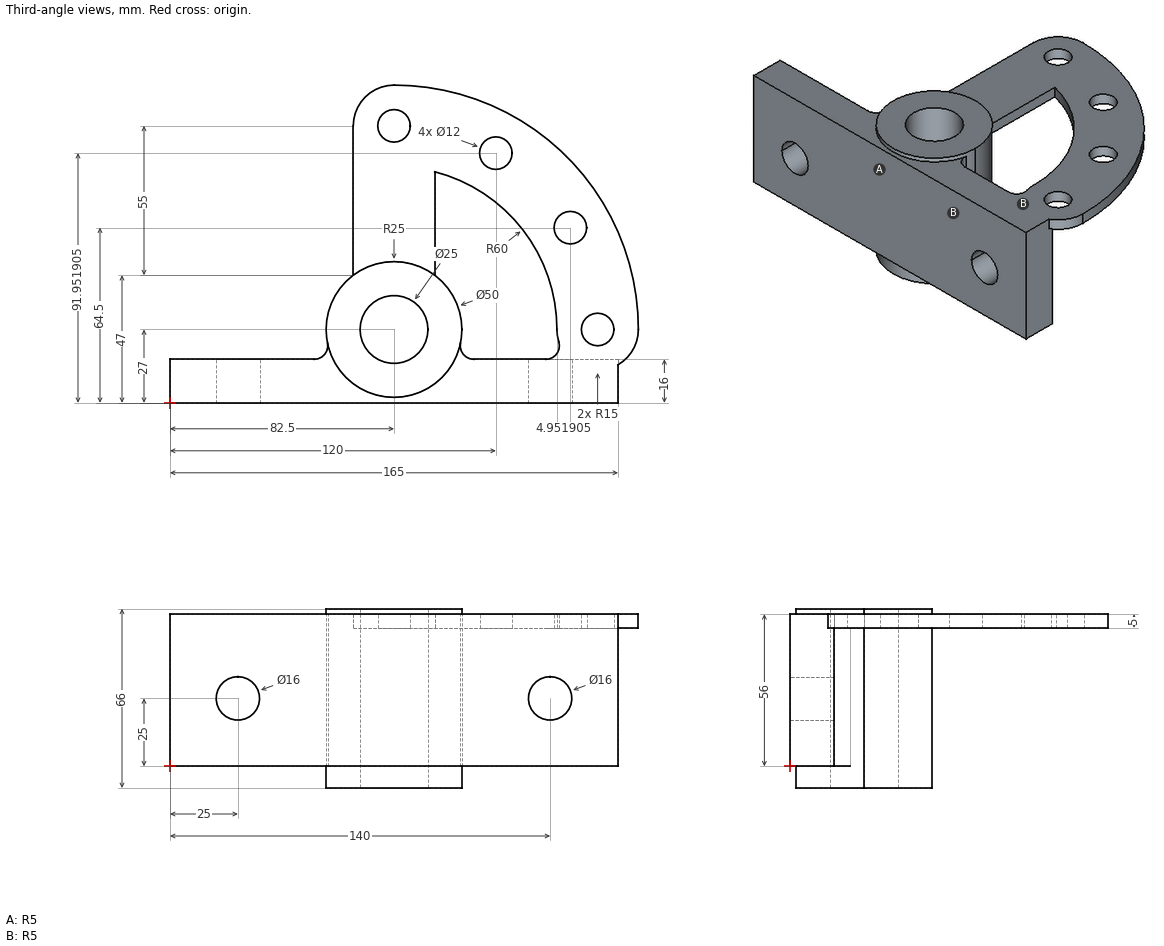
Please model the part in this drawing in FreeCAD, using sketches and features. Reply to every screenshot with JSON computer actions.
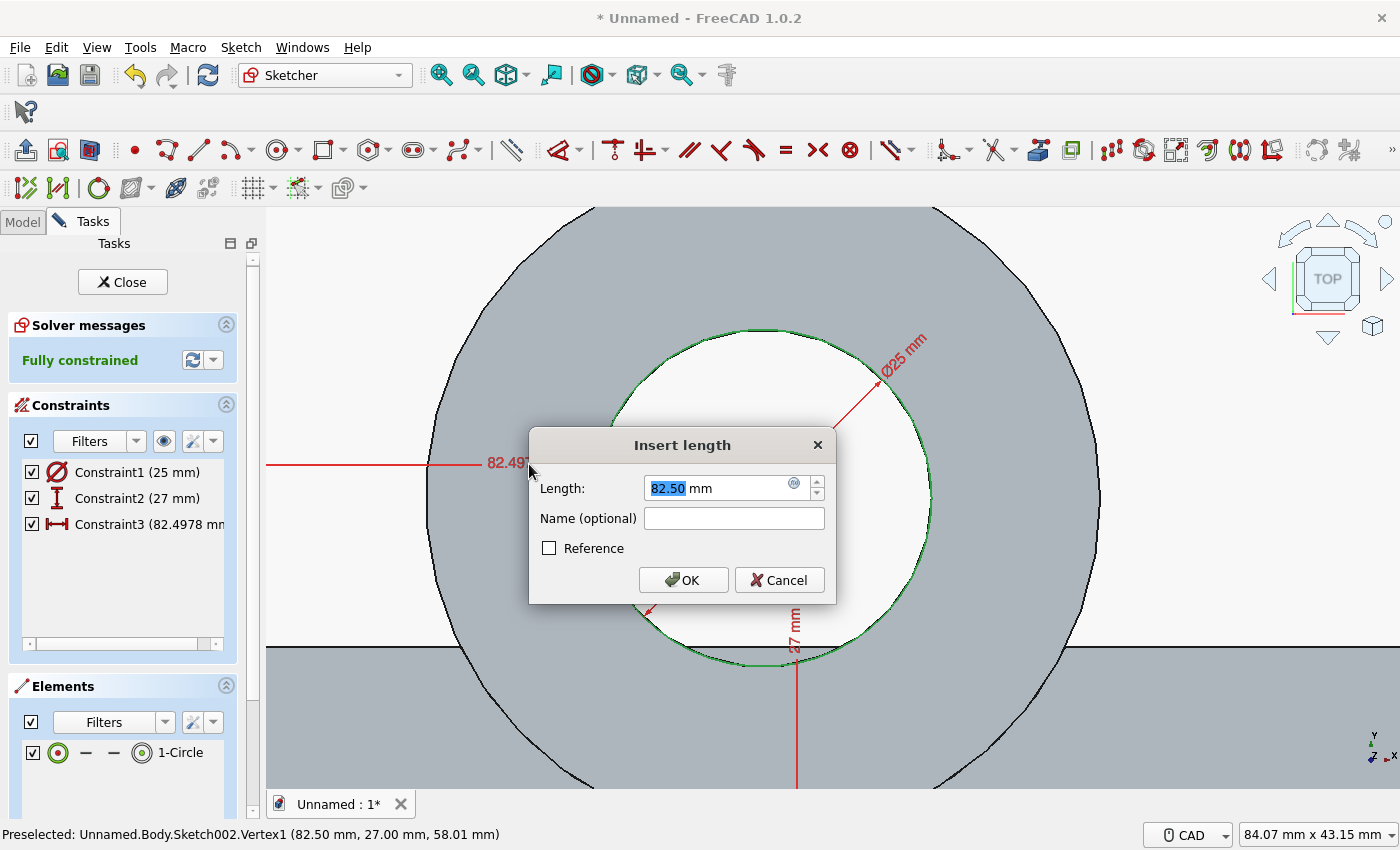
{"action": "type", "text": "82.5"}
{"action": "key", "text": "Return"}
{"action": "key", "text": "Escape"}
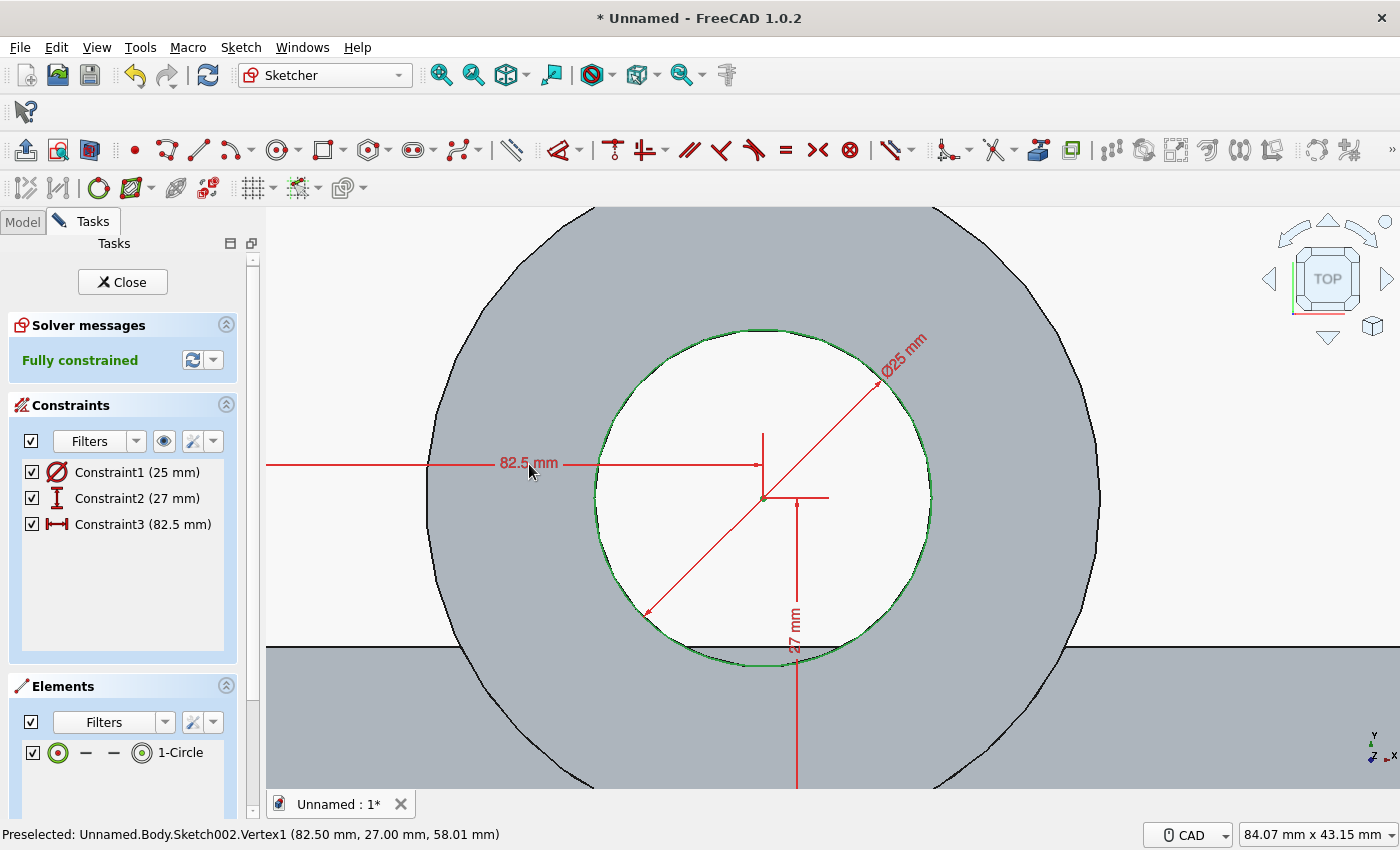
{"action": "left_click", "coordinate": [123, 282]}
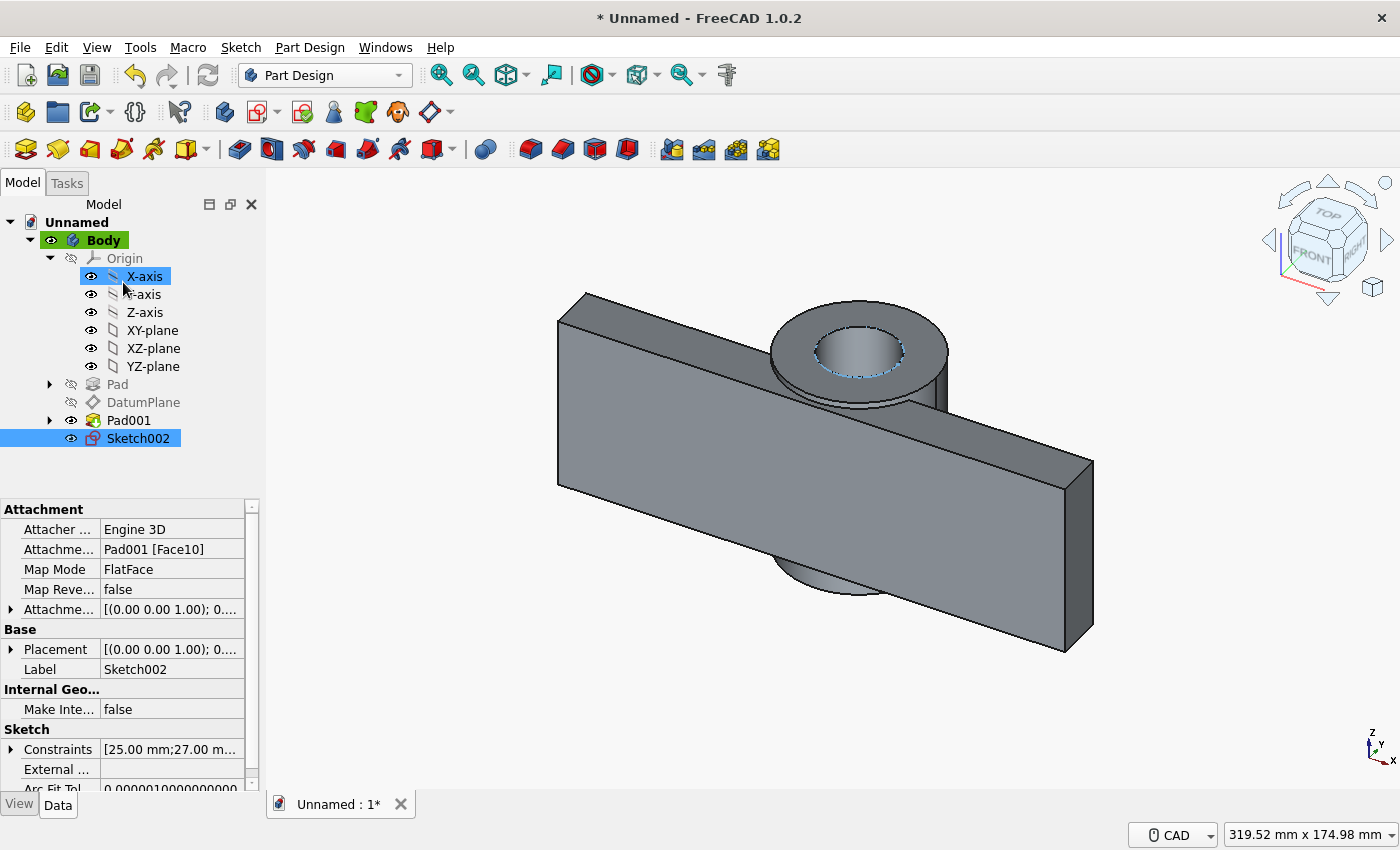
{"action": "left_click", "coordinate": [240, 150]}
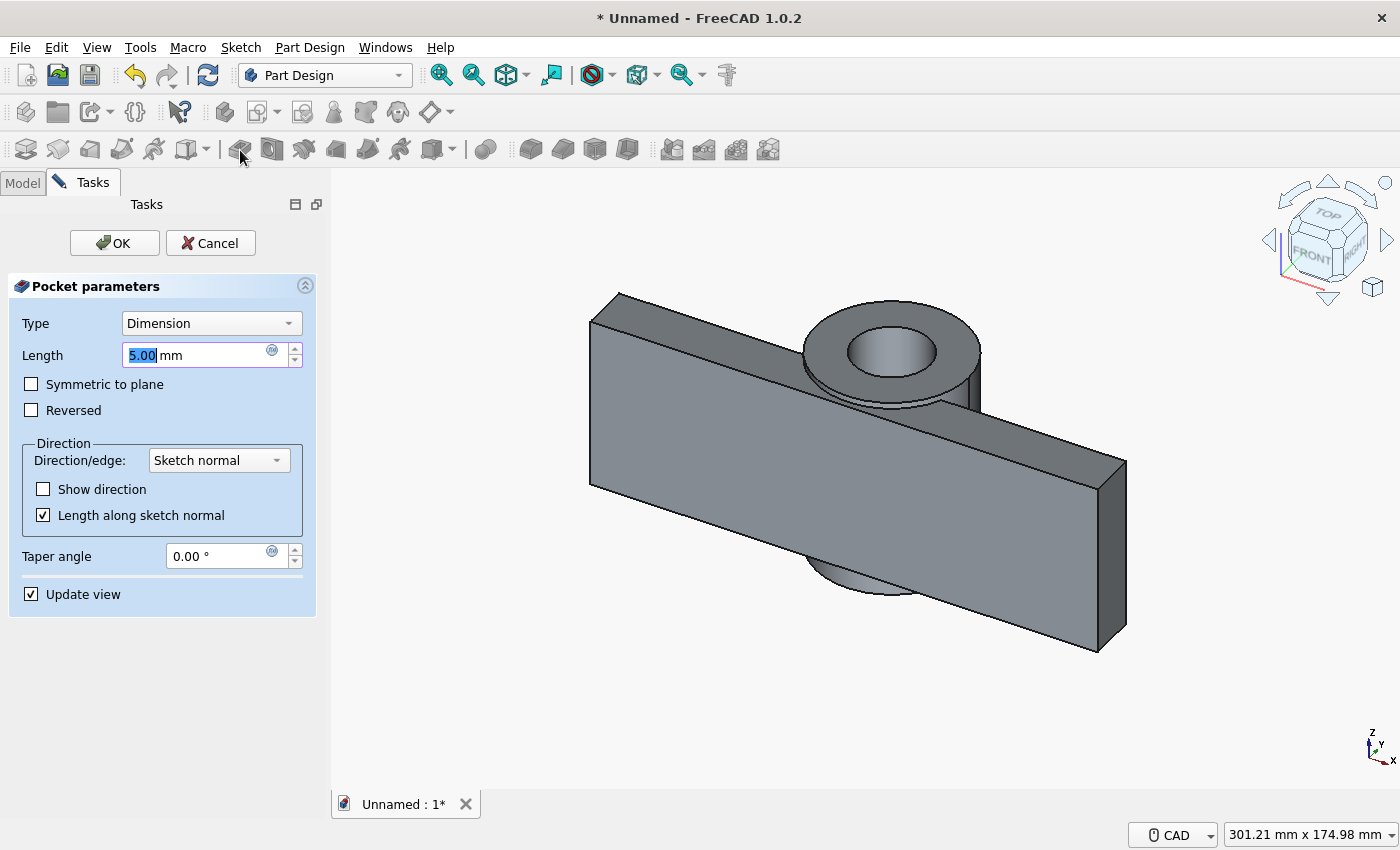
{"action": "left_click", "coordinate": [212, 324]}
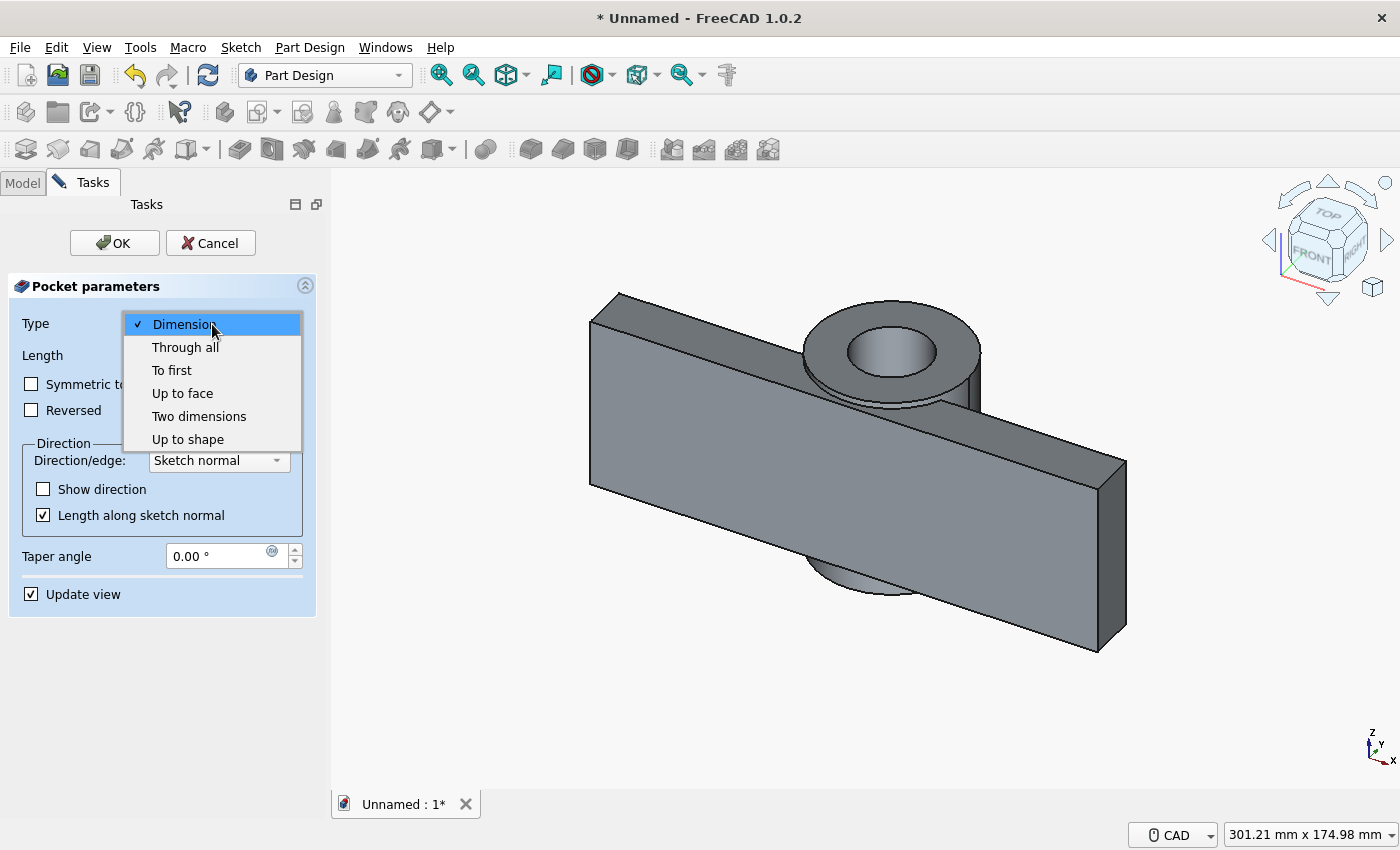
{"action": "left_click", "coordinate": [212, 348]}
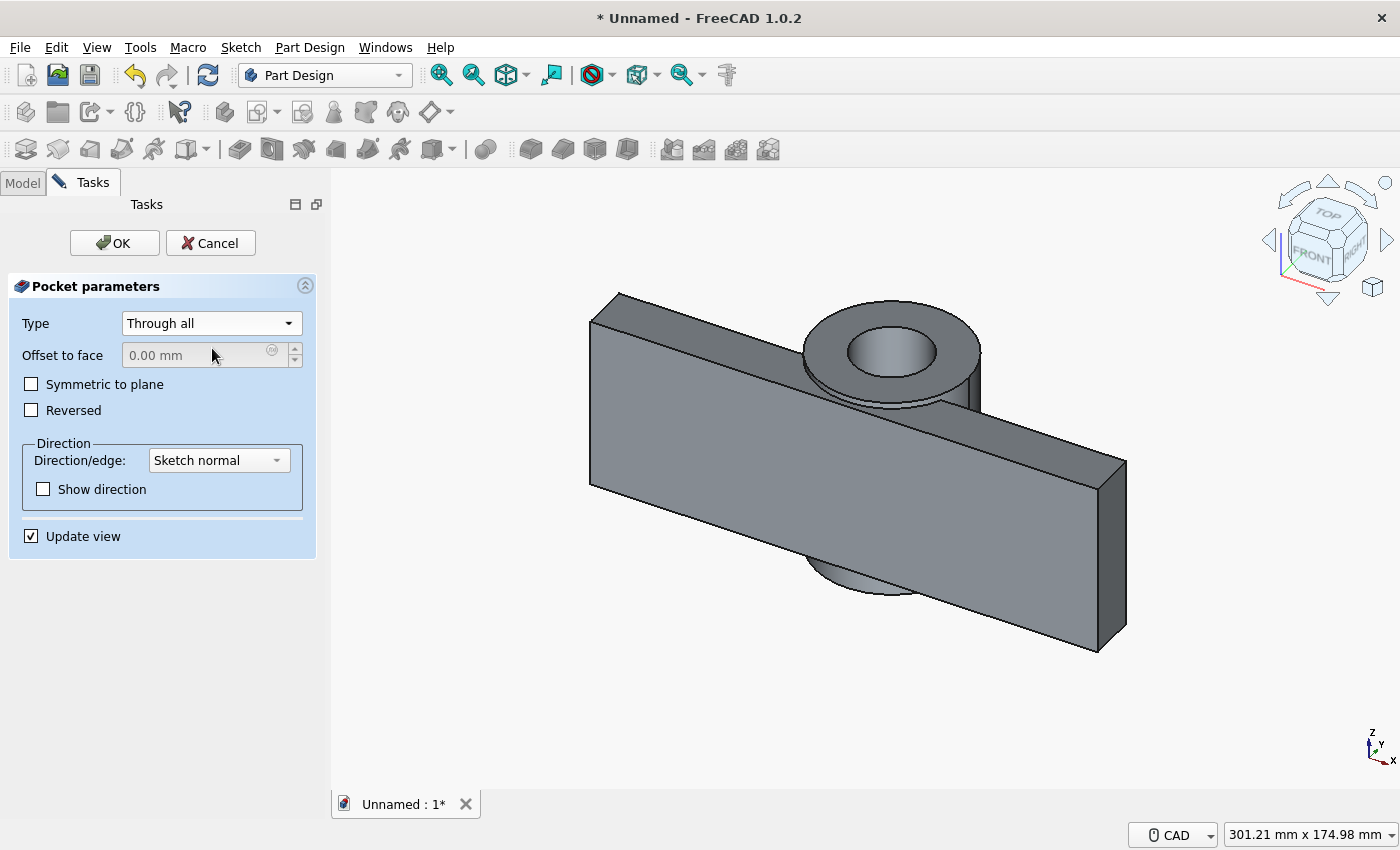
{"action": "left_click", "coordinate": [115, 243]}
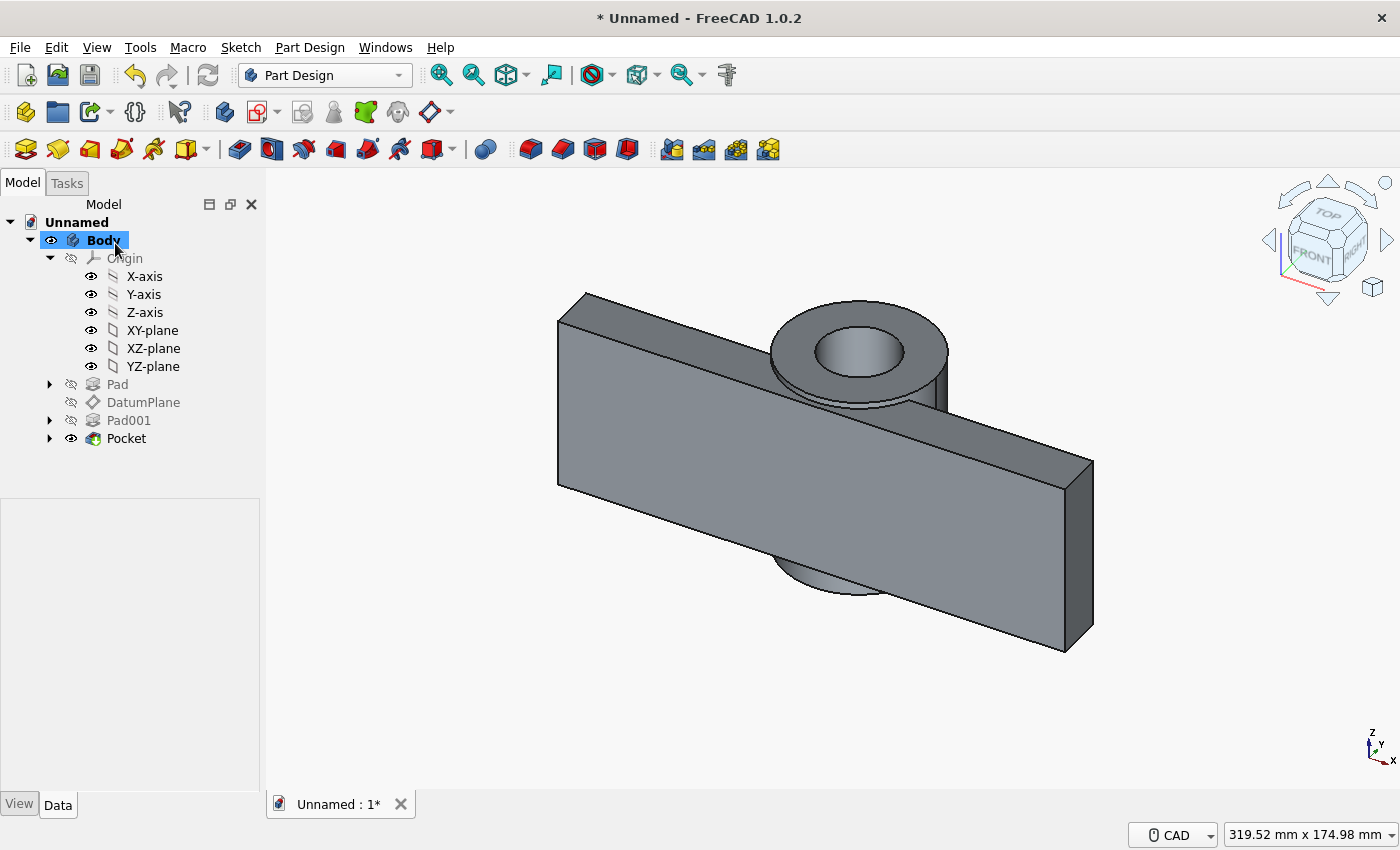
{"action": "left_click", "coordinate": [1043, 462]}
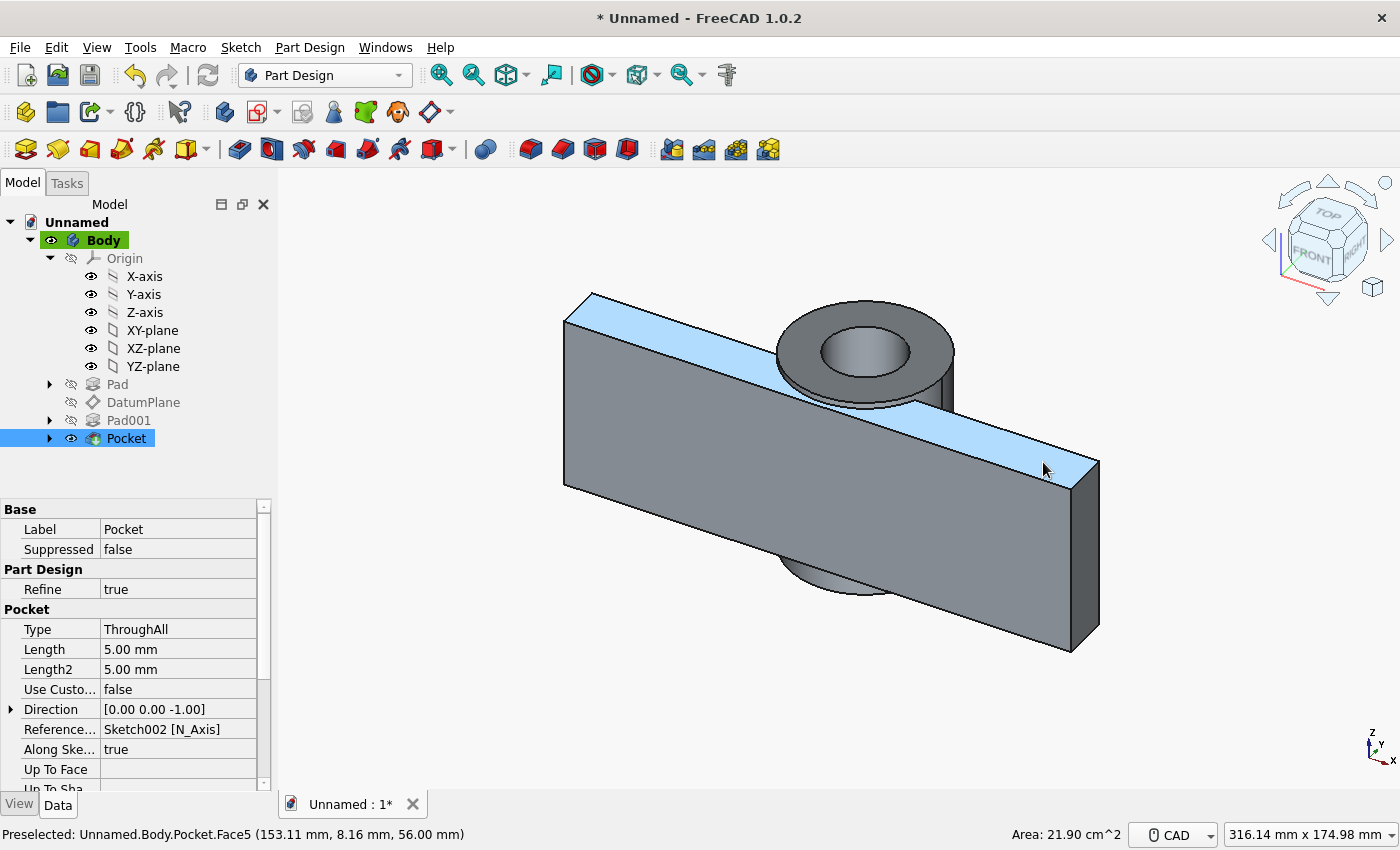
{"action": "left_click", "coordinate": [258, 112]}